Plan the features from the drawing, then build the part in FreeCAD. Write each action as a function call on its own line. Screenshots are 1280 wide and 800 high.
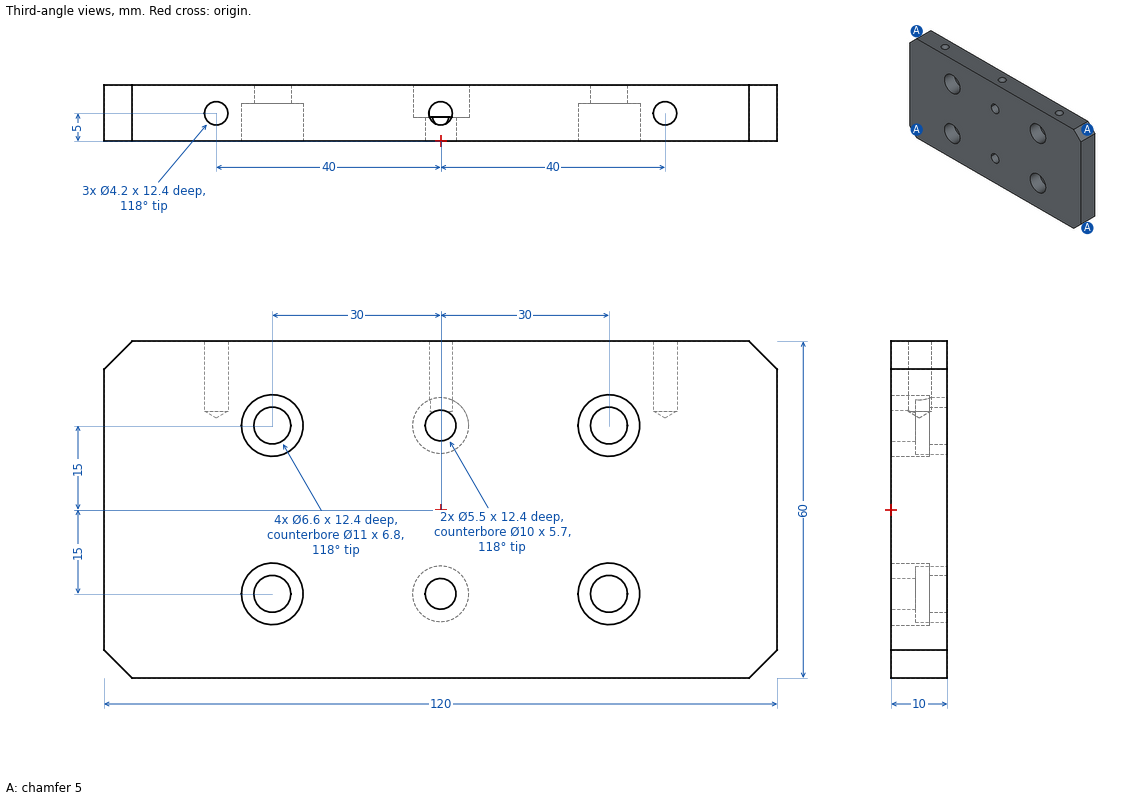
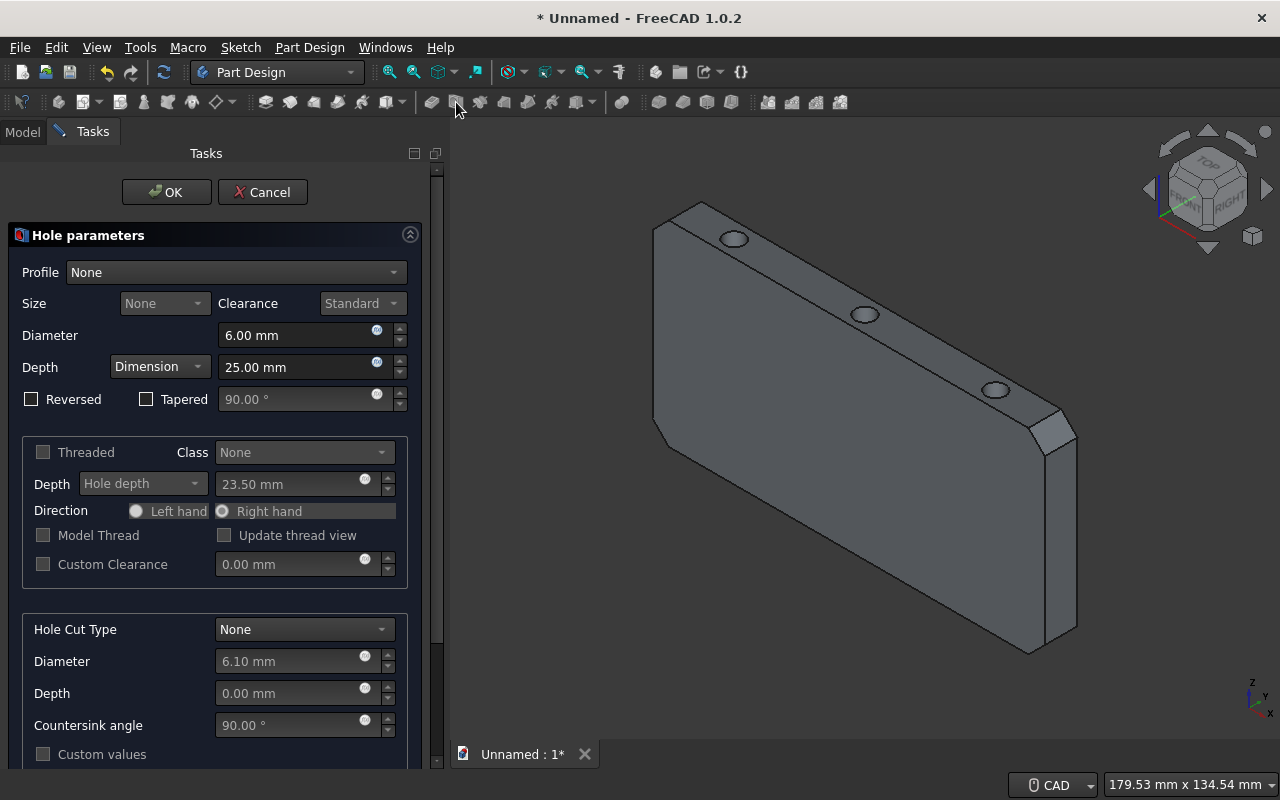
triple_click(305, 335)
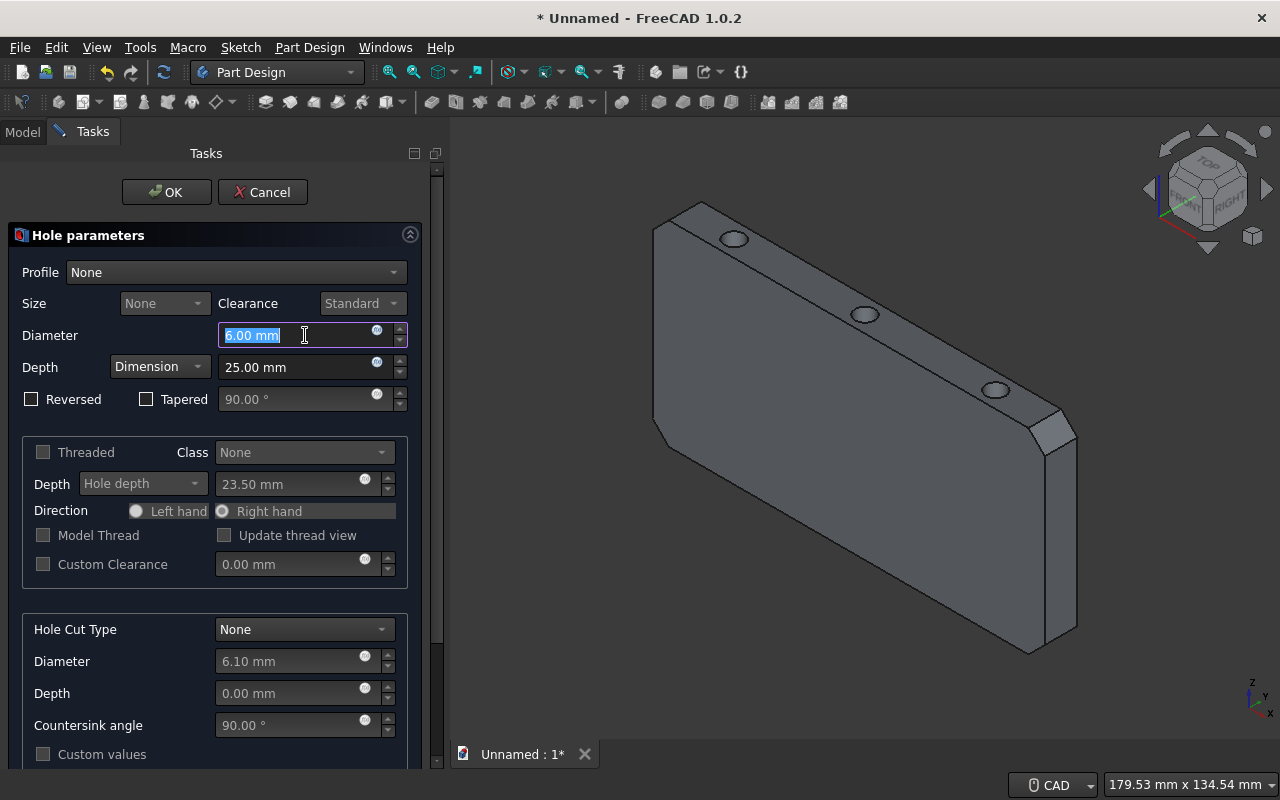
text(4.2)
key(Tab)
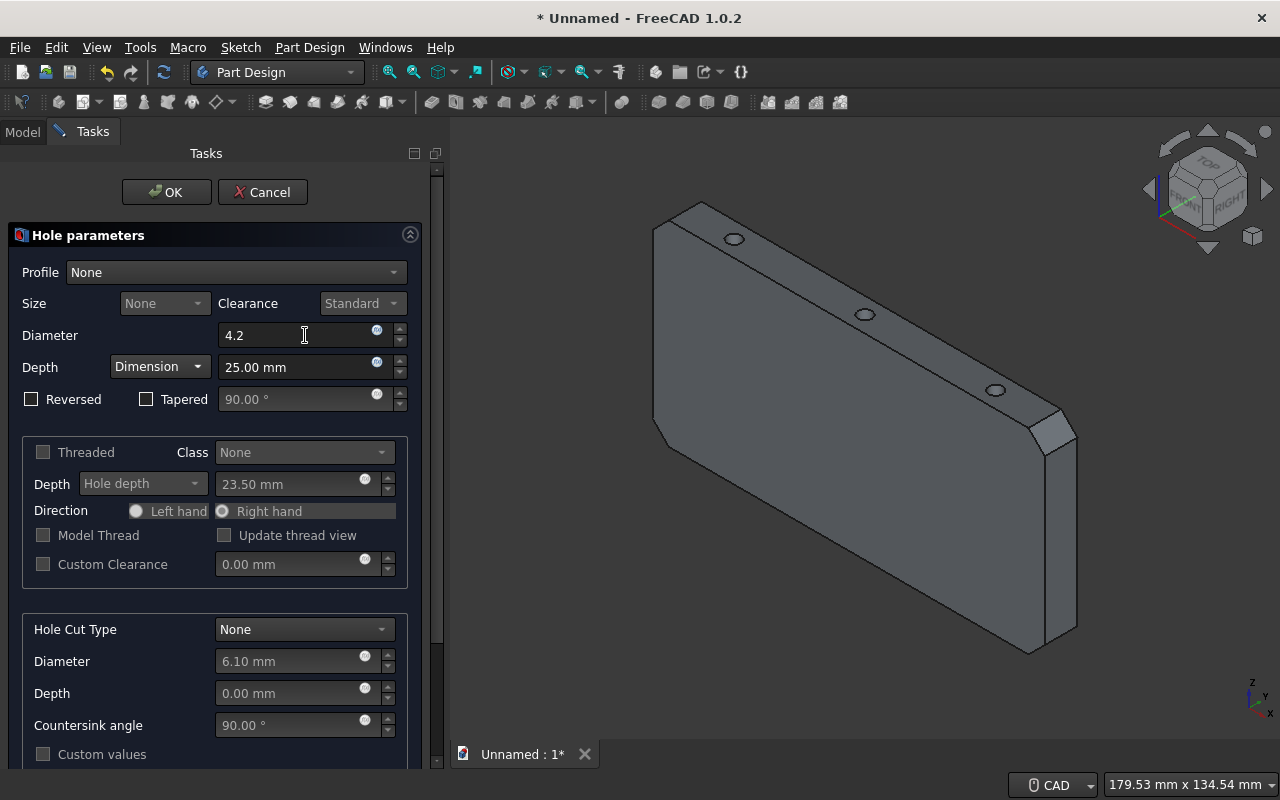
triple_click(305, 367)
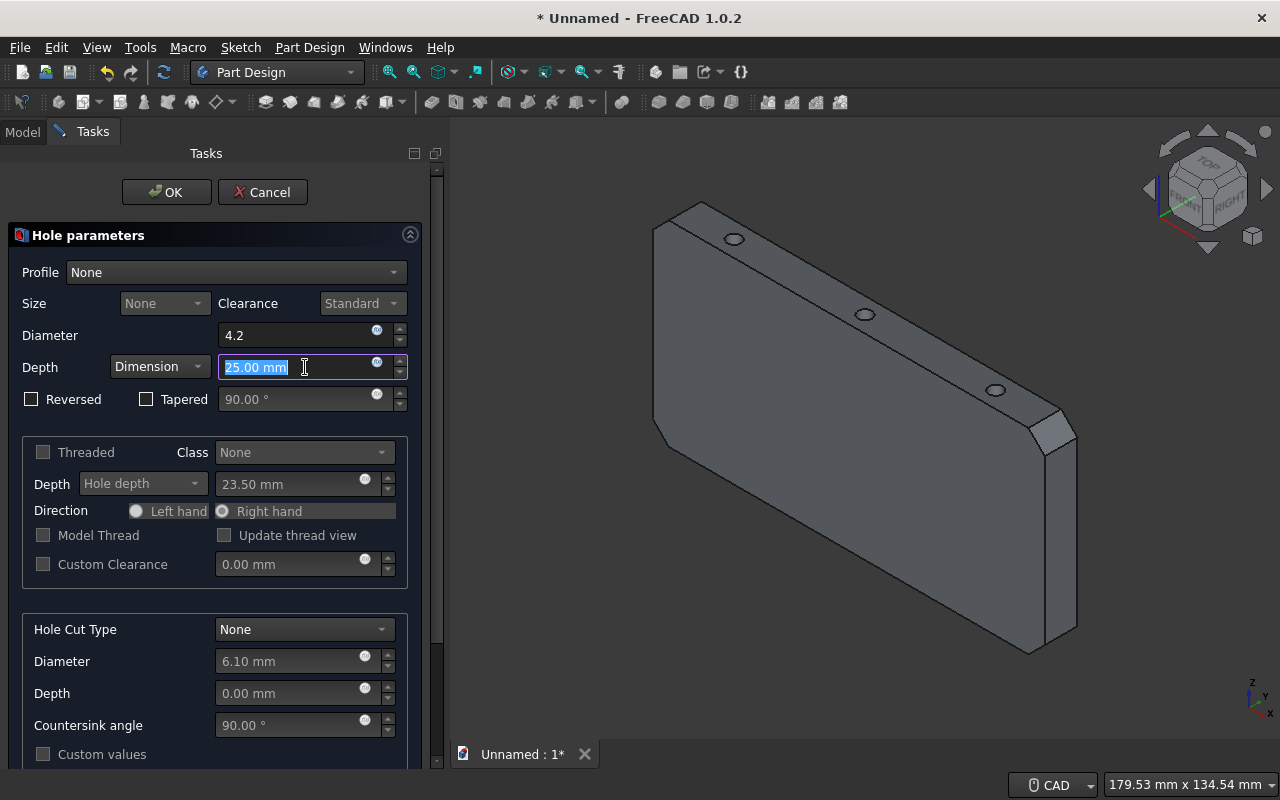
text(12.4)
key(Tab)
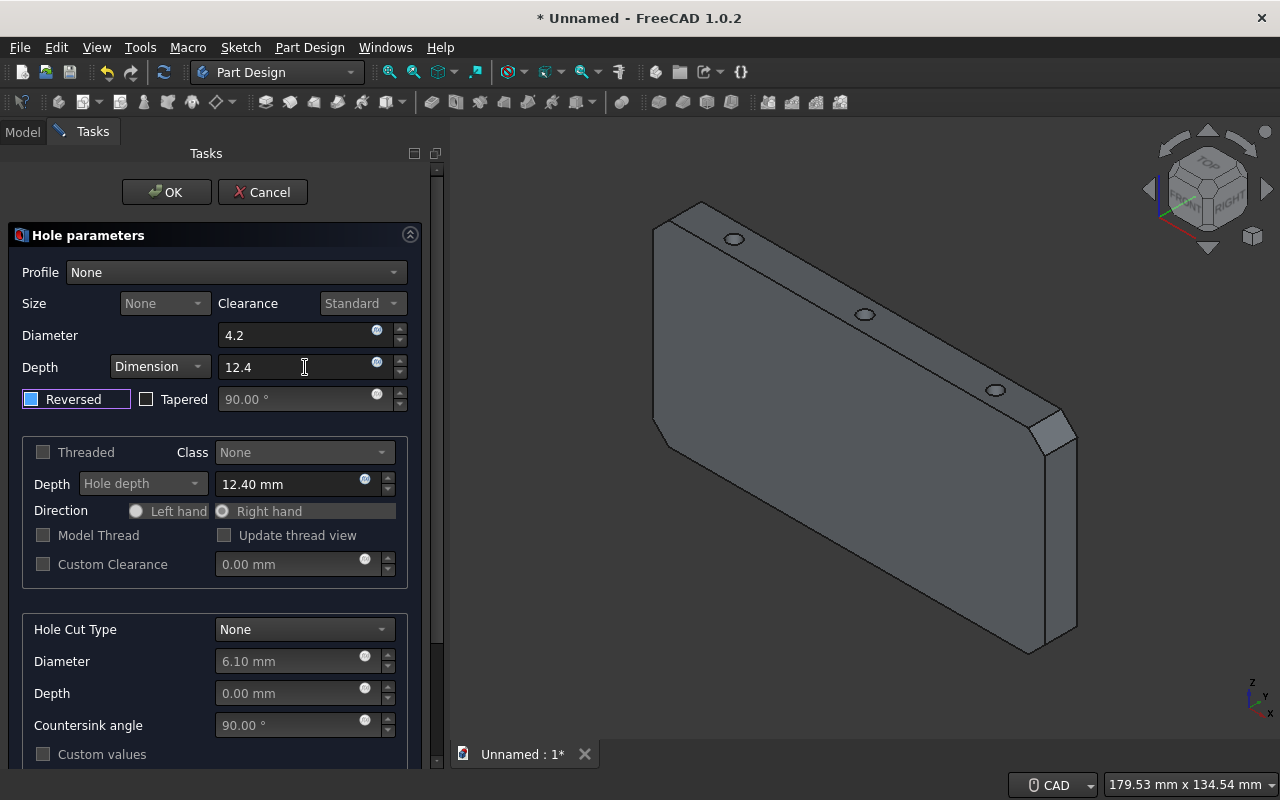
click(167, 192)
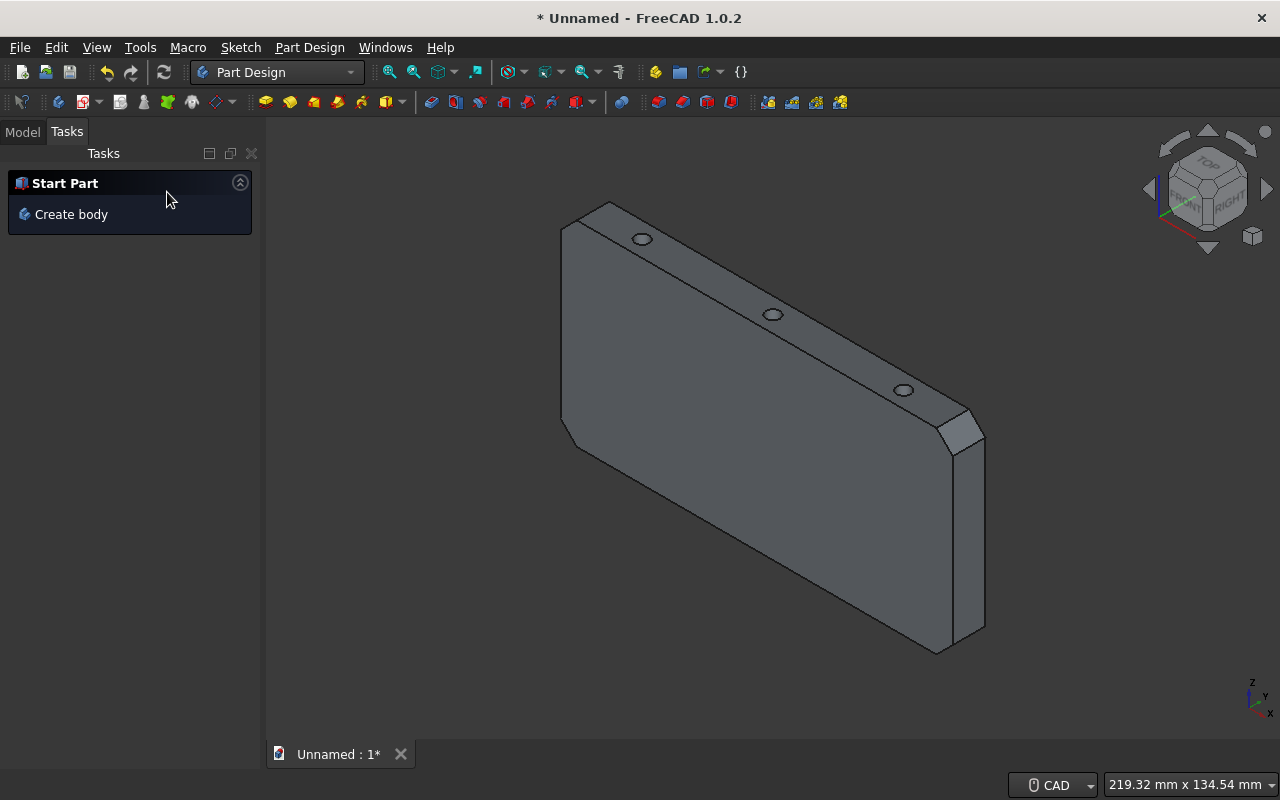
click(813, 469)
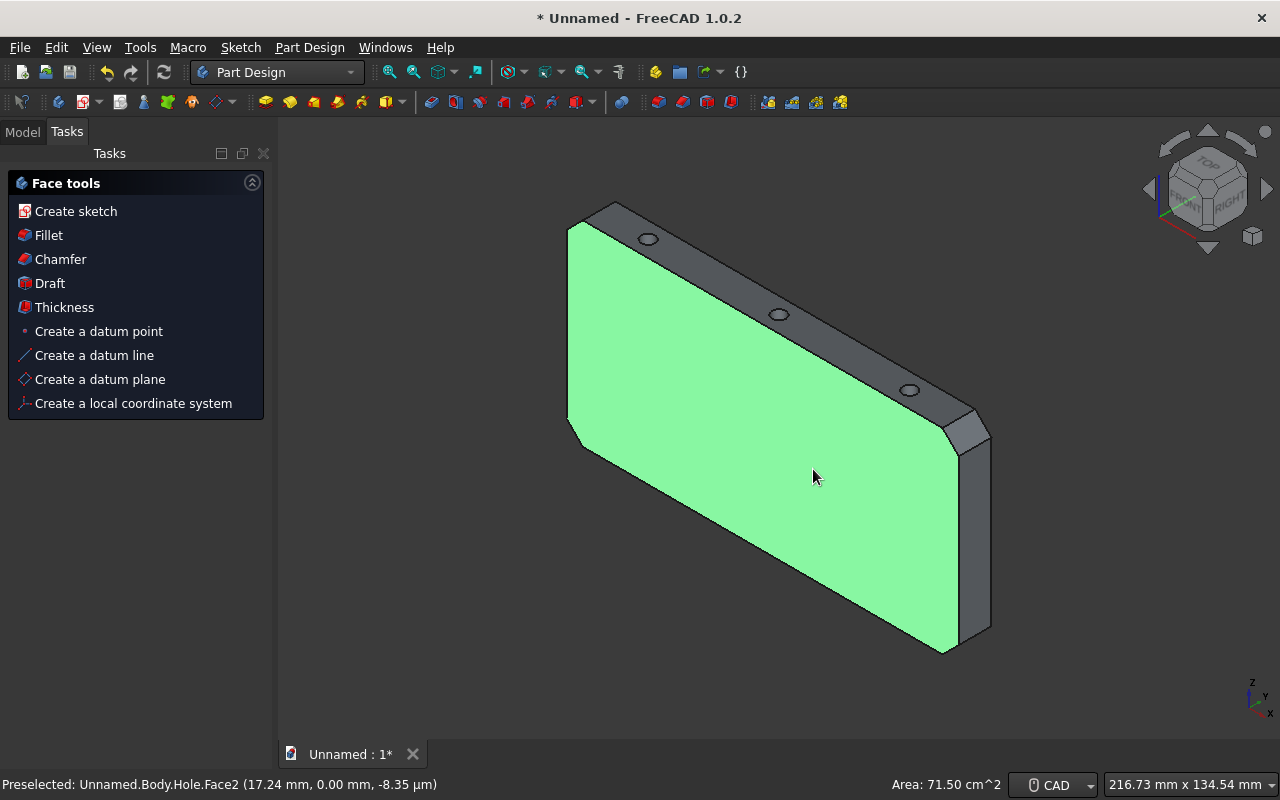
click(84, 102)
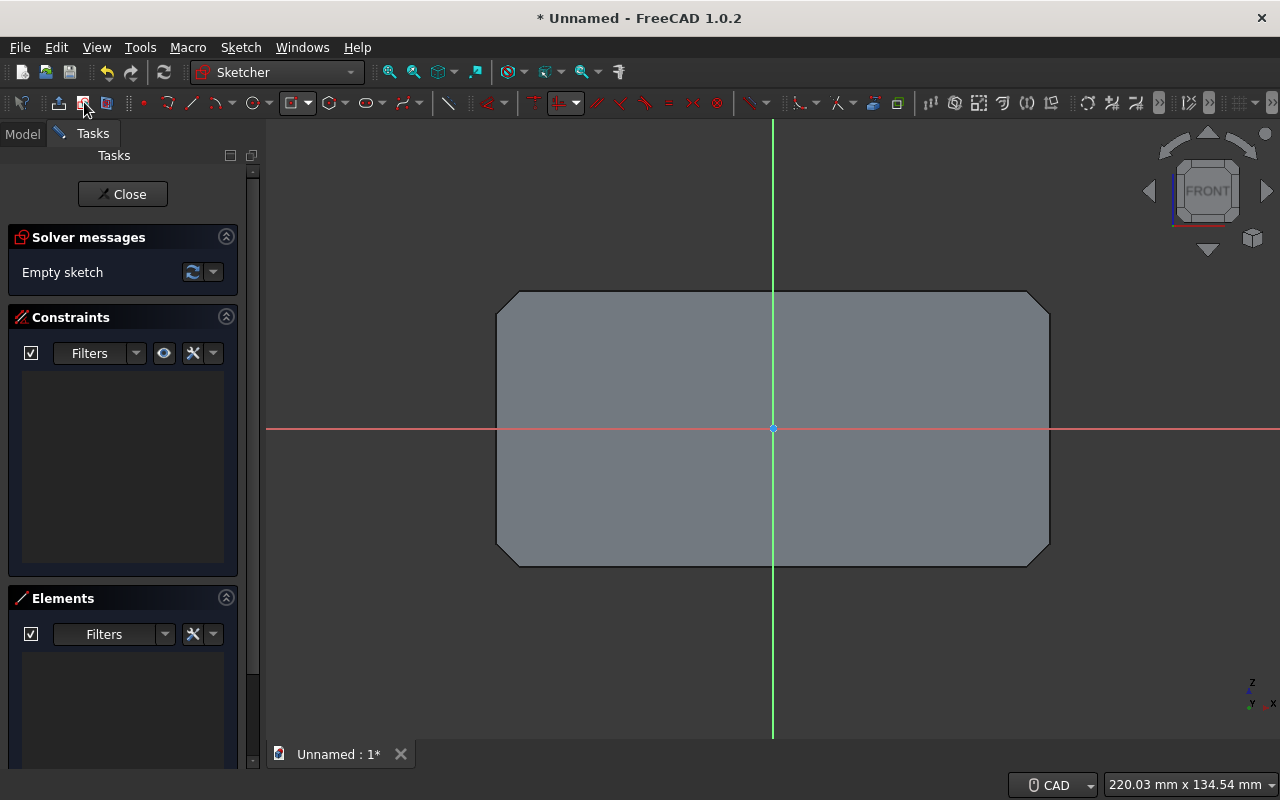
scroll(856, 429, up, 3)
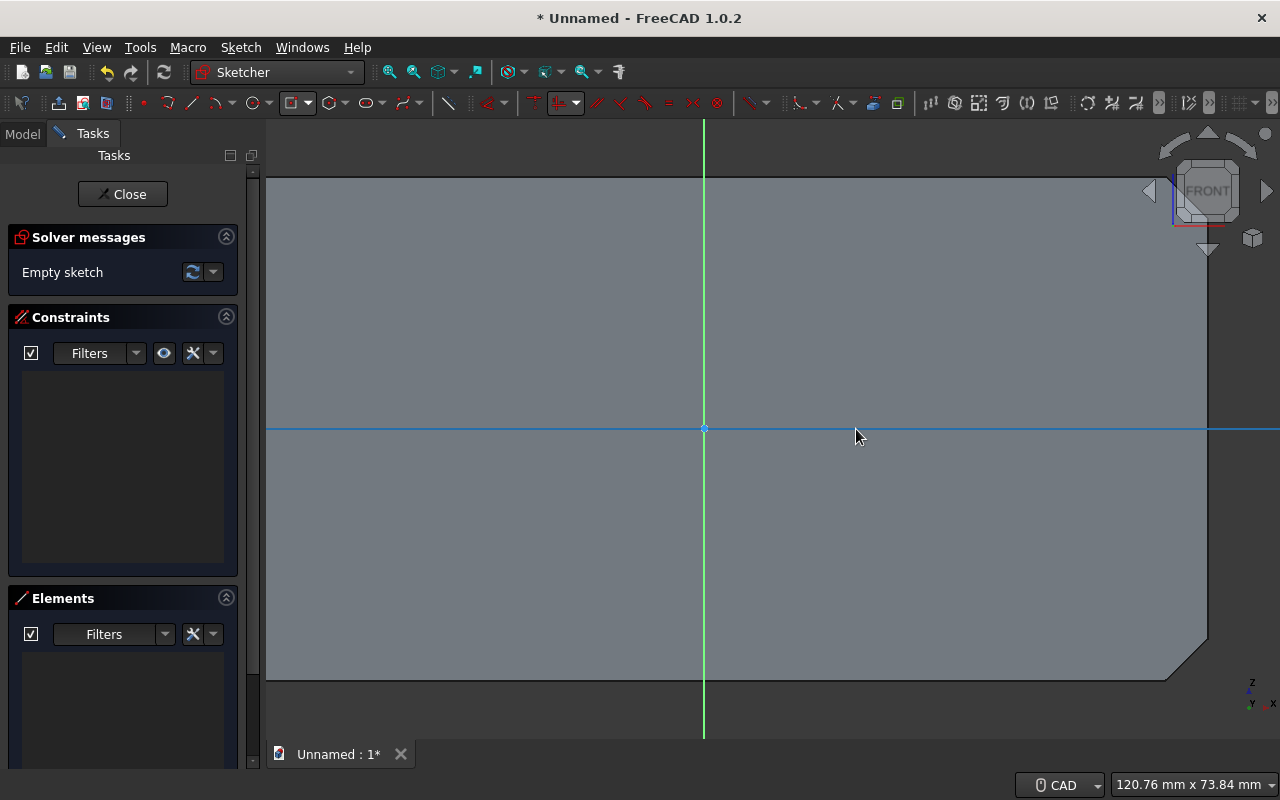
key(g)
key(c)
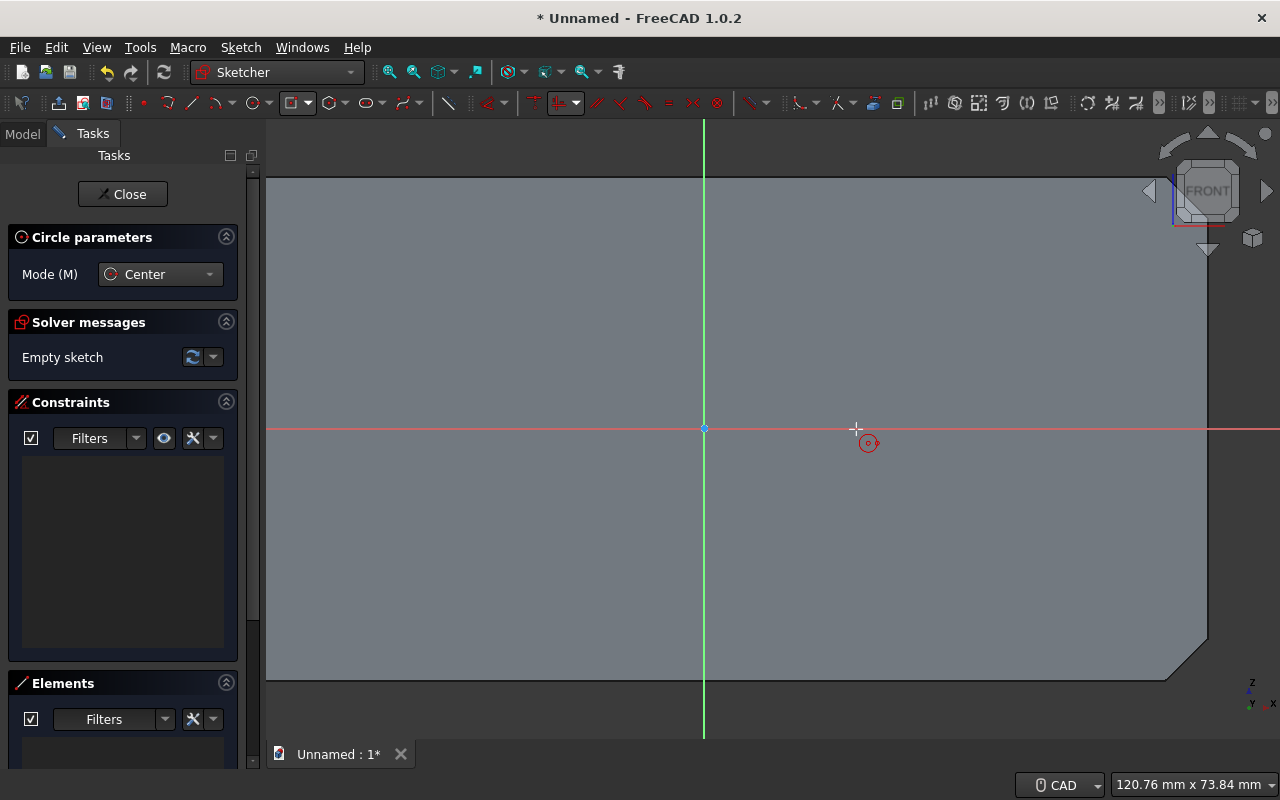
click(452, 303)
move(472, 283)